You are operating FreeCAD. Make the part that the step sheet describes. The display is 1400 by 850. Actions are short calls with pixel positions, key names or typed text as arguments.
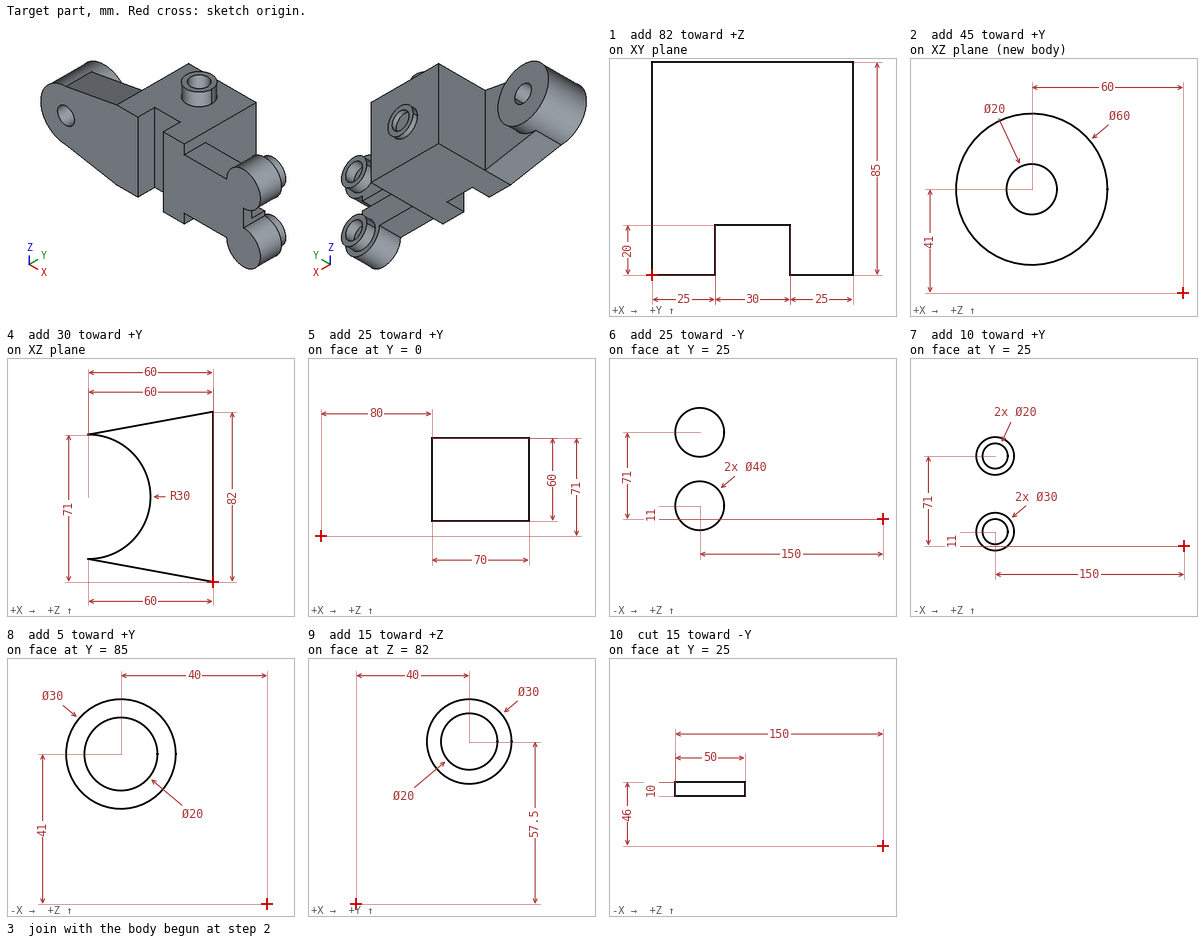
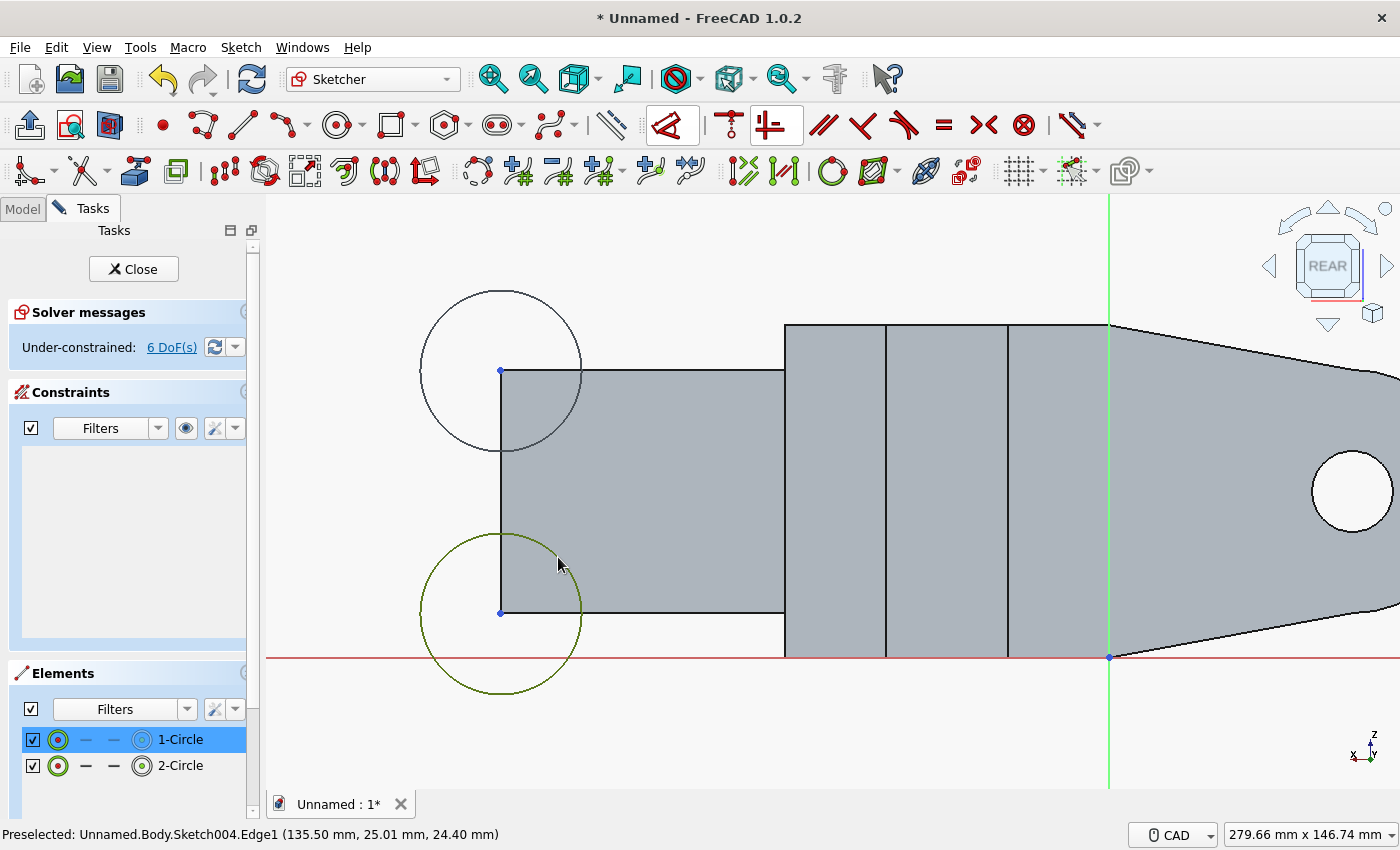
click(558, 314)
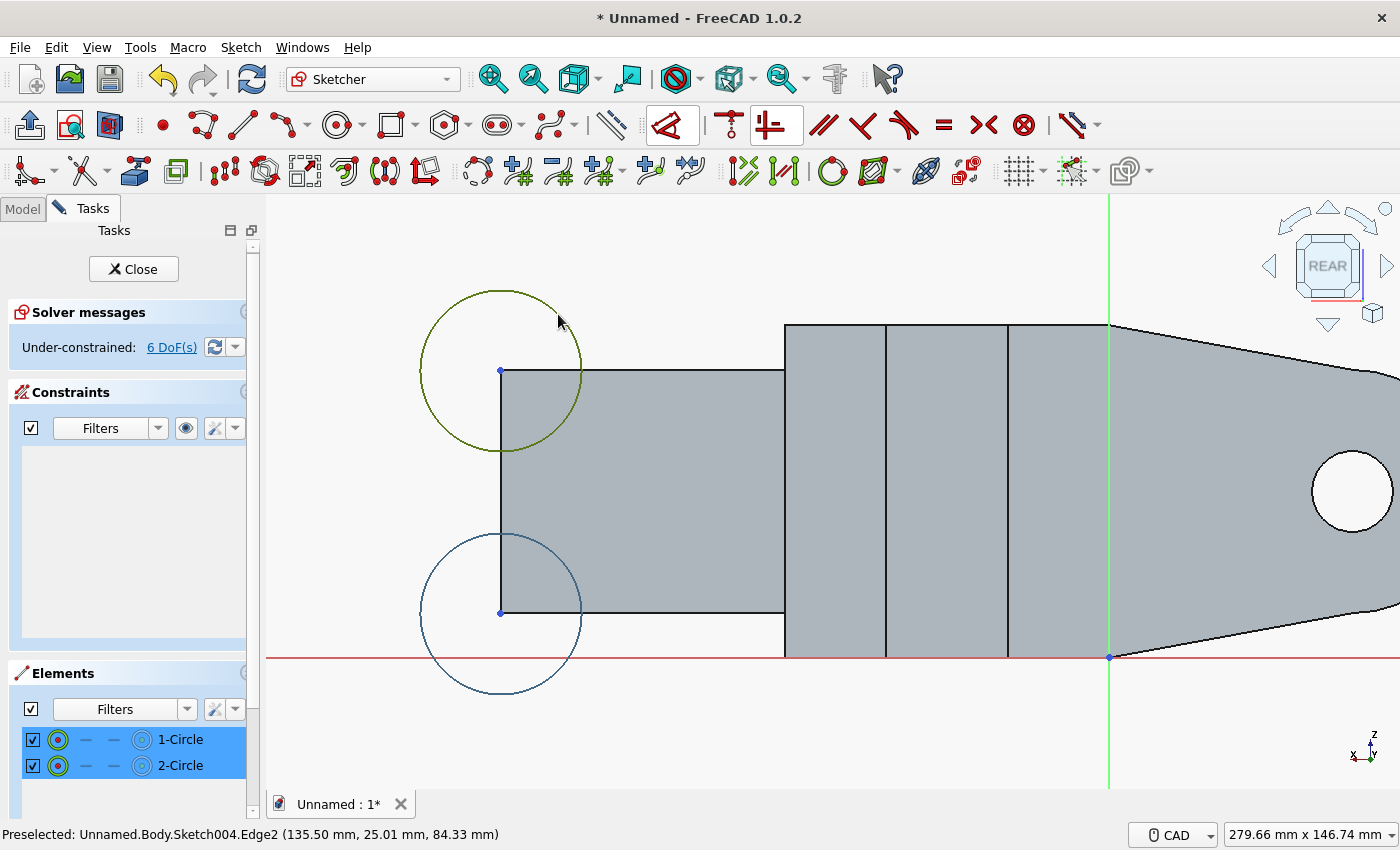
click(944, 126)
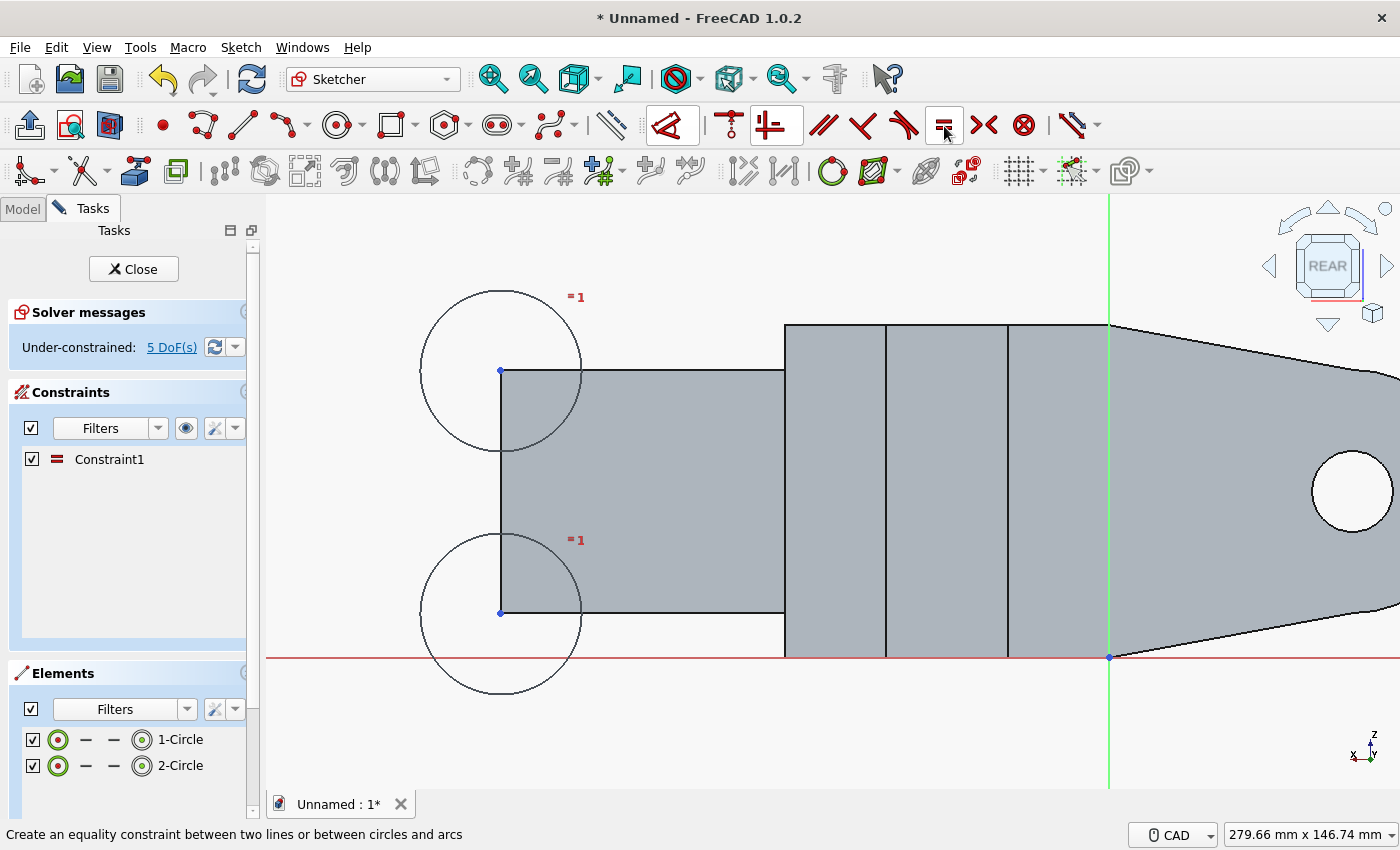
click(501, 614)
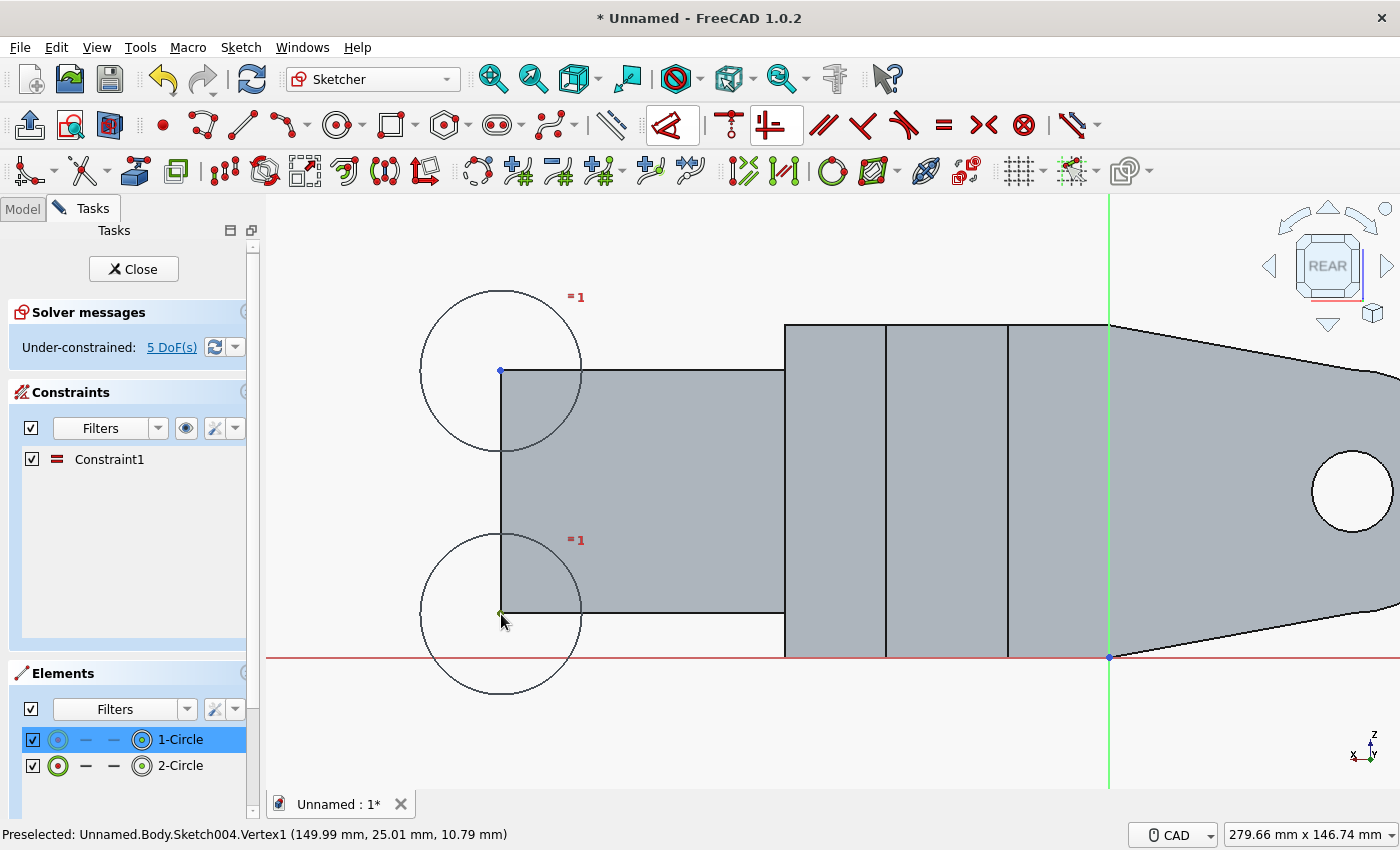
click(501, 371)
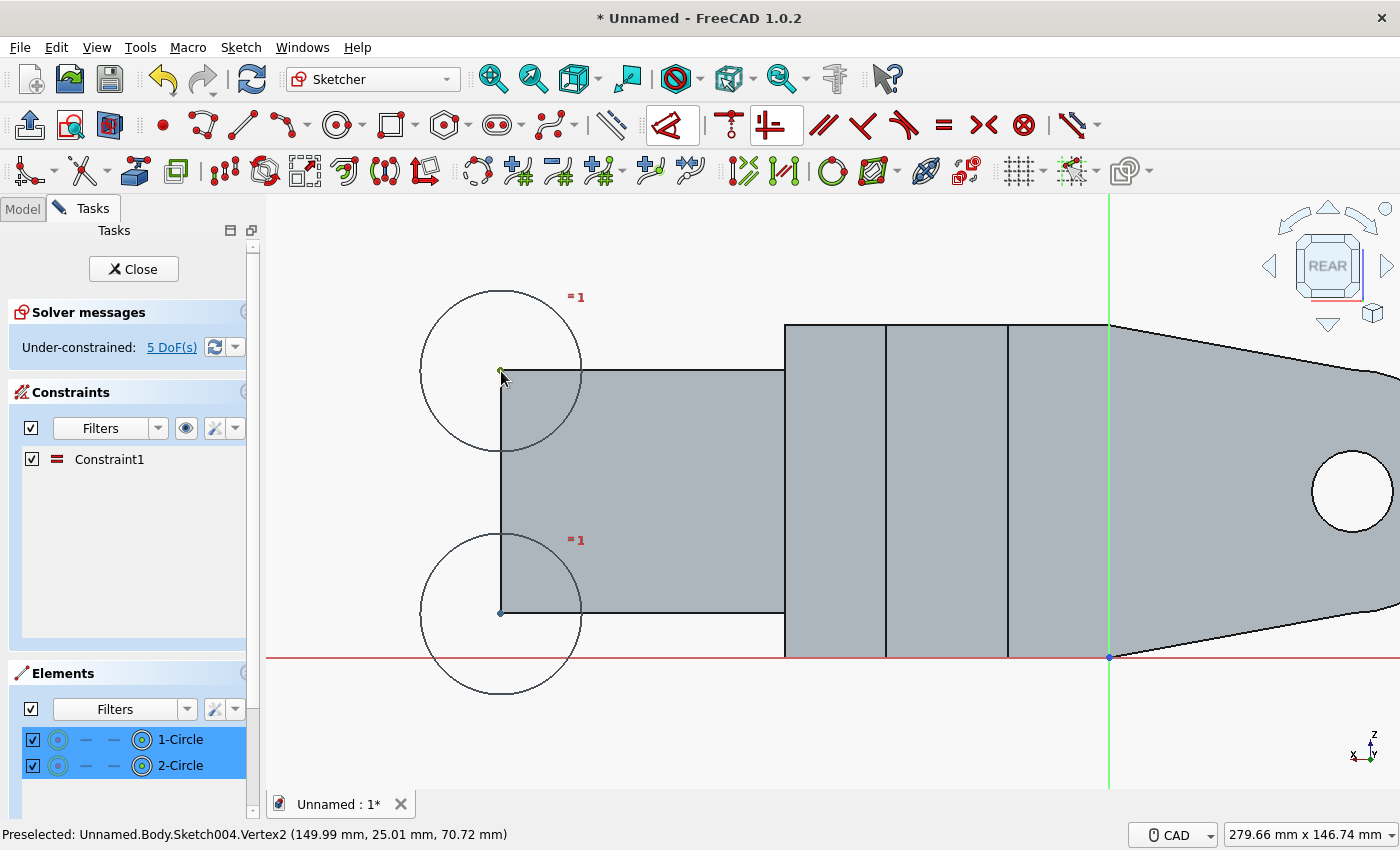
click(798, 126)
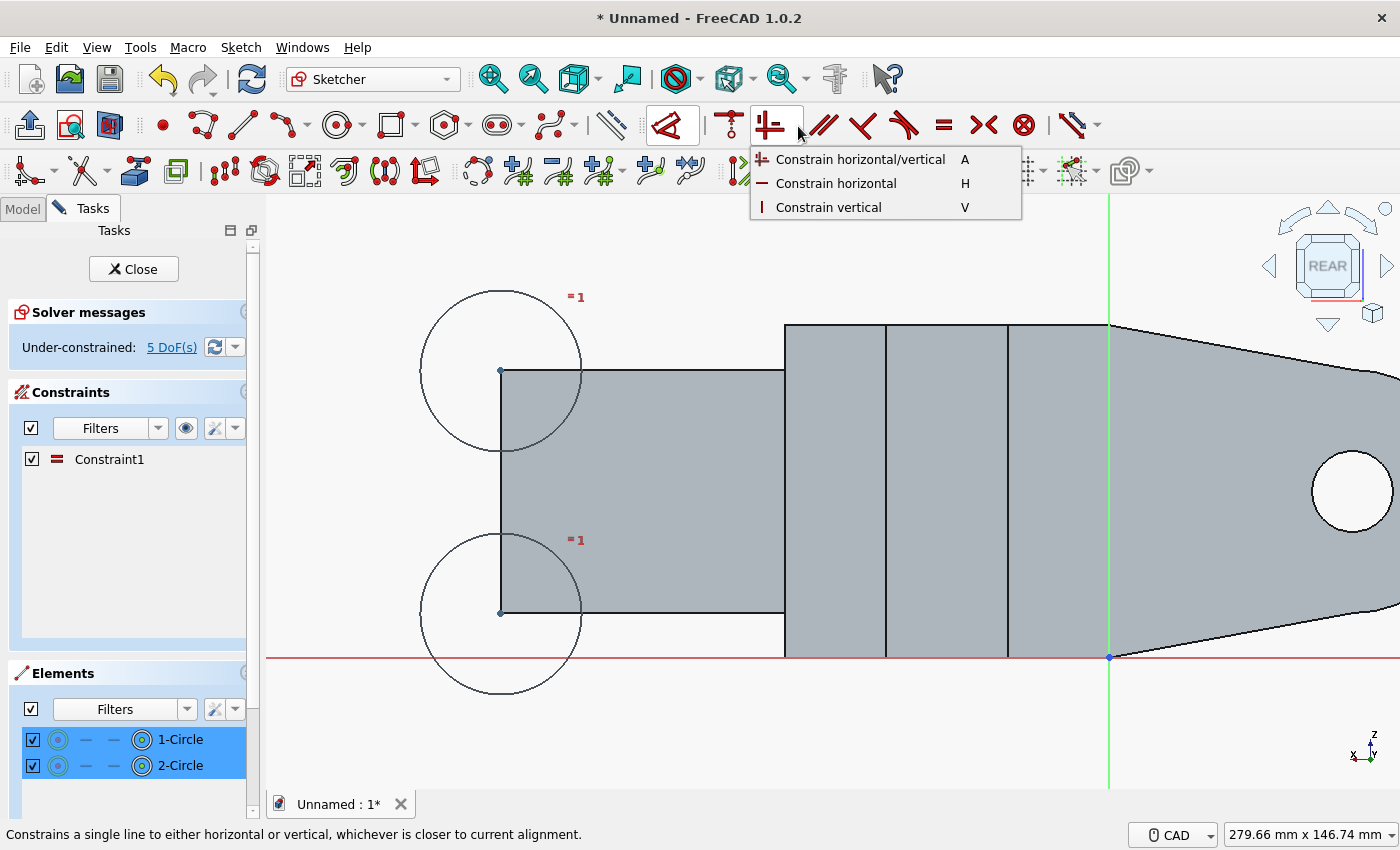
click(886, 207)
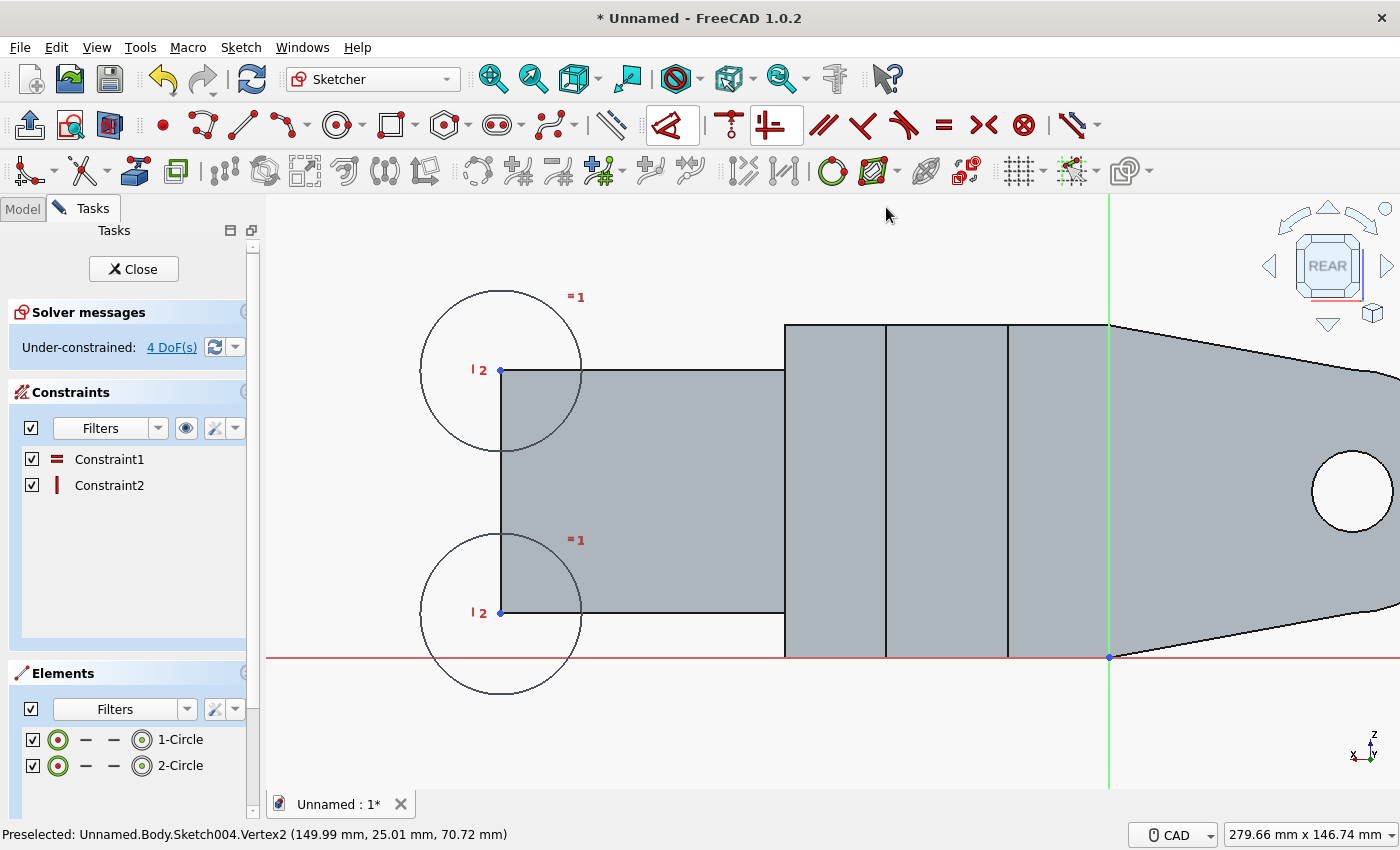
click(558, 557)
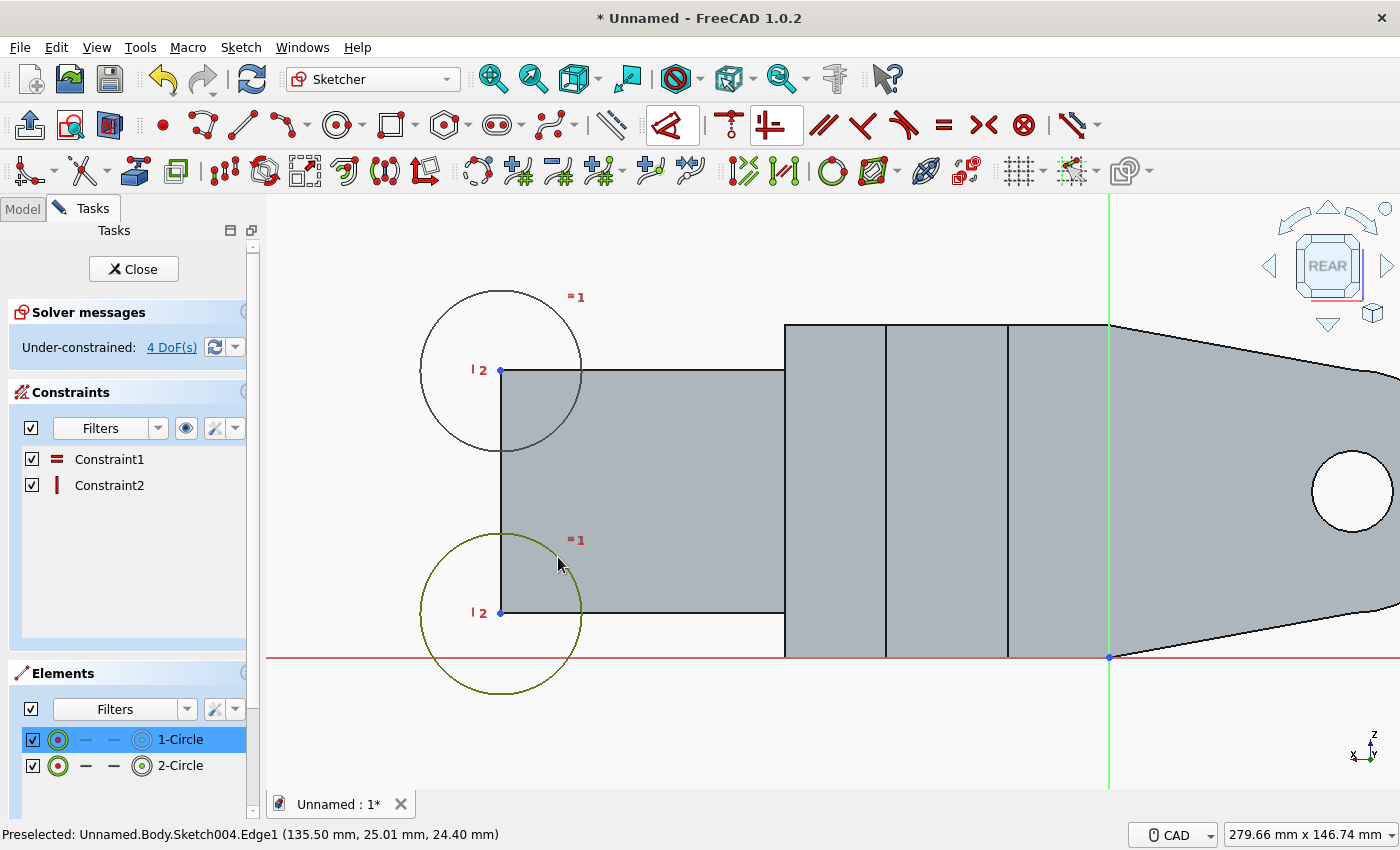
key(k)
key(o)